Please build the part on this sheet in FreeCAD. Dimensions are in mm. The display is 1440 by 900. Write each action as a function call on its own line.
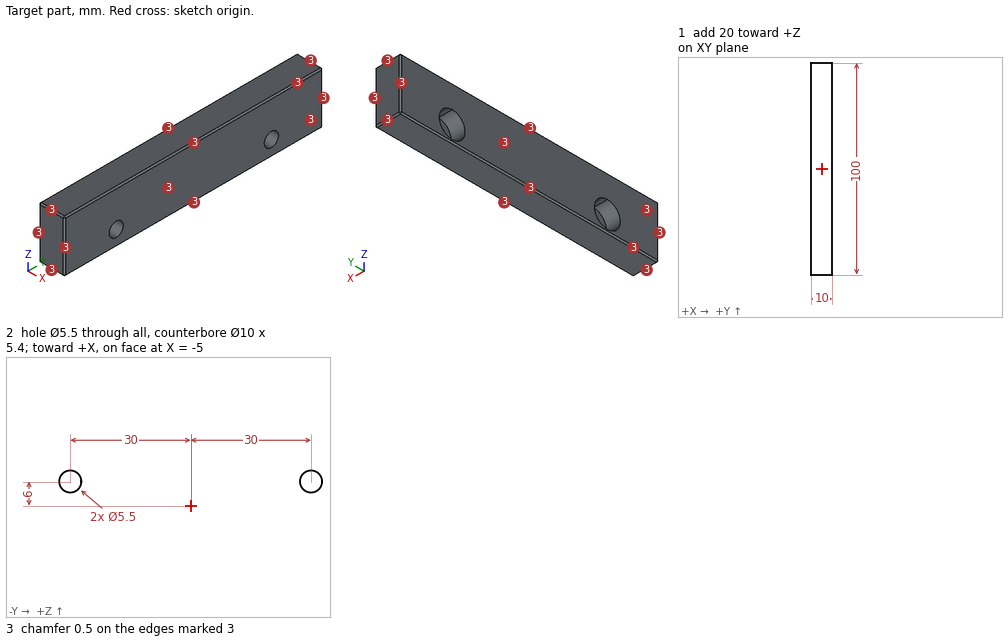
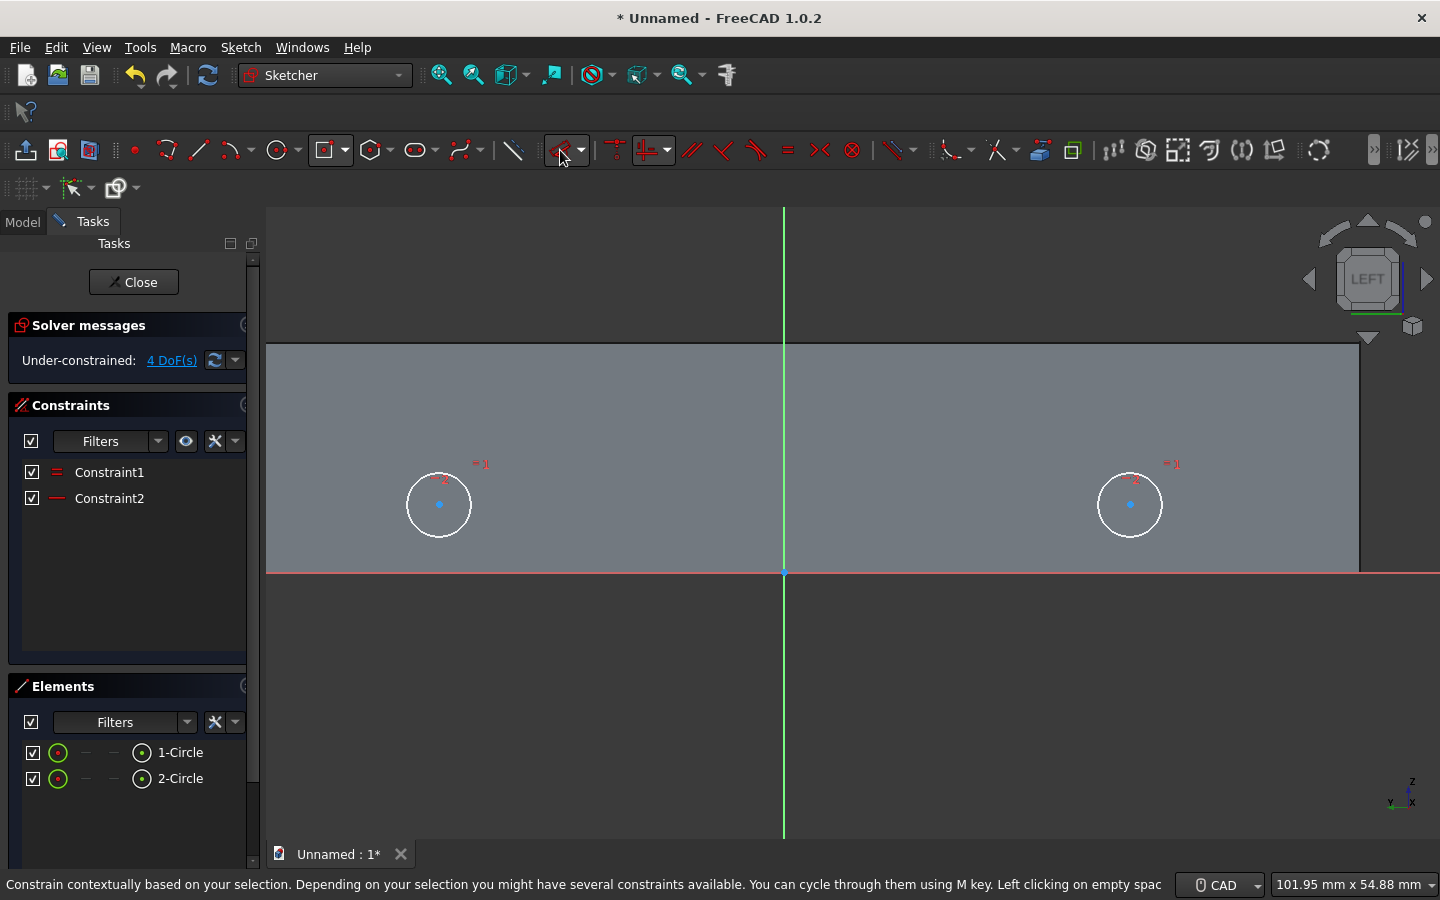
click(461, 482)
click(483, 459)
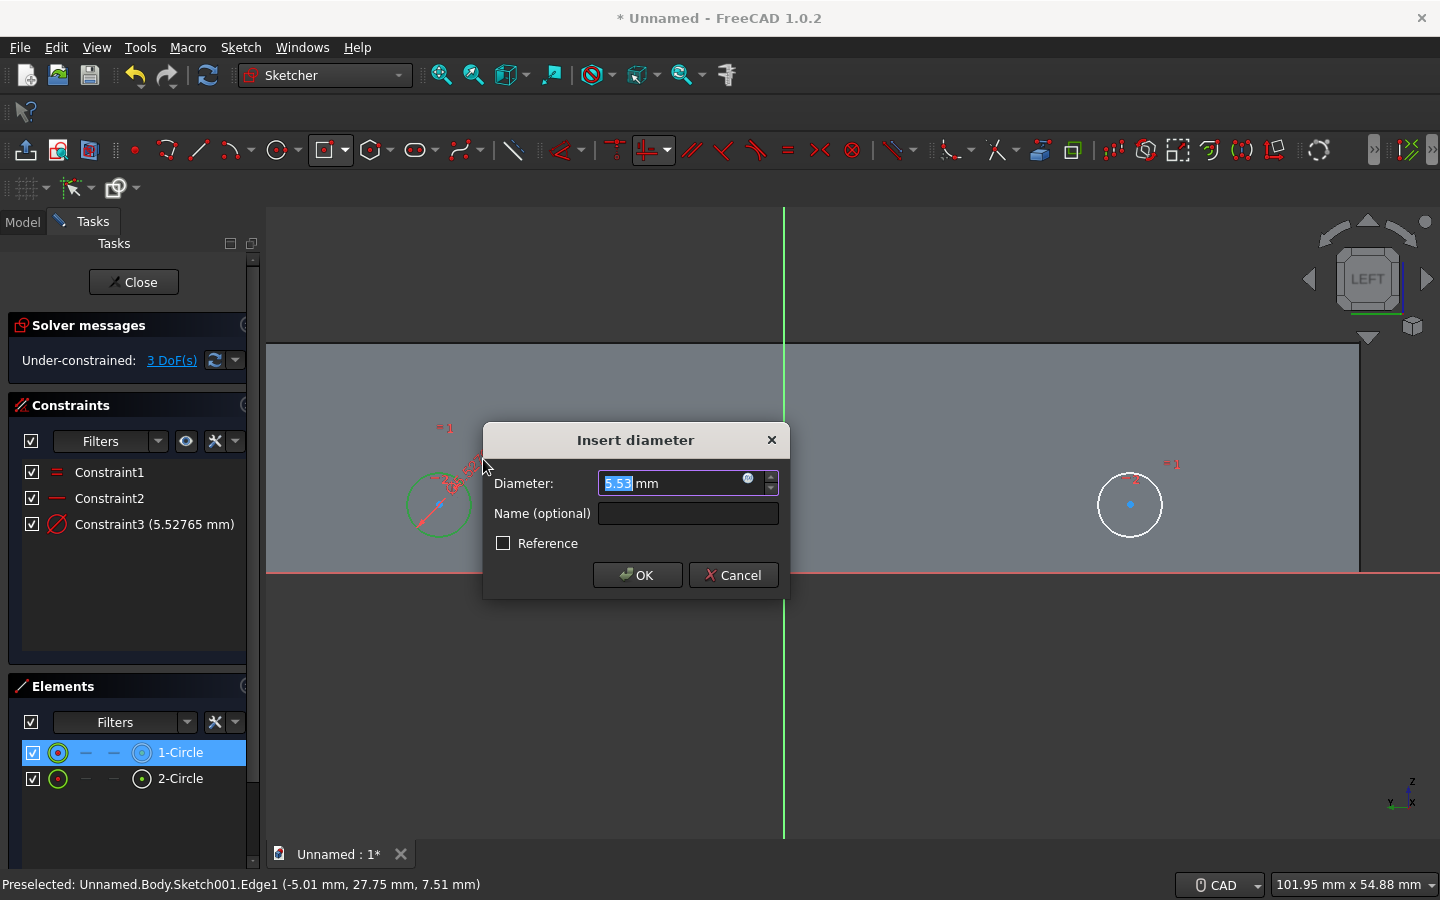
text(5.5)
key(Return)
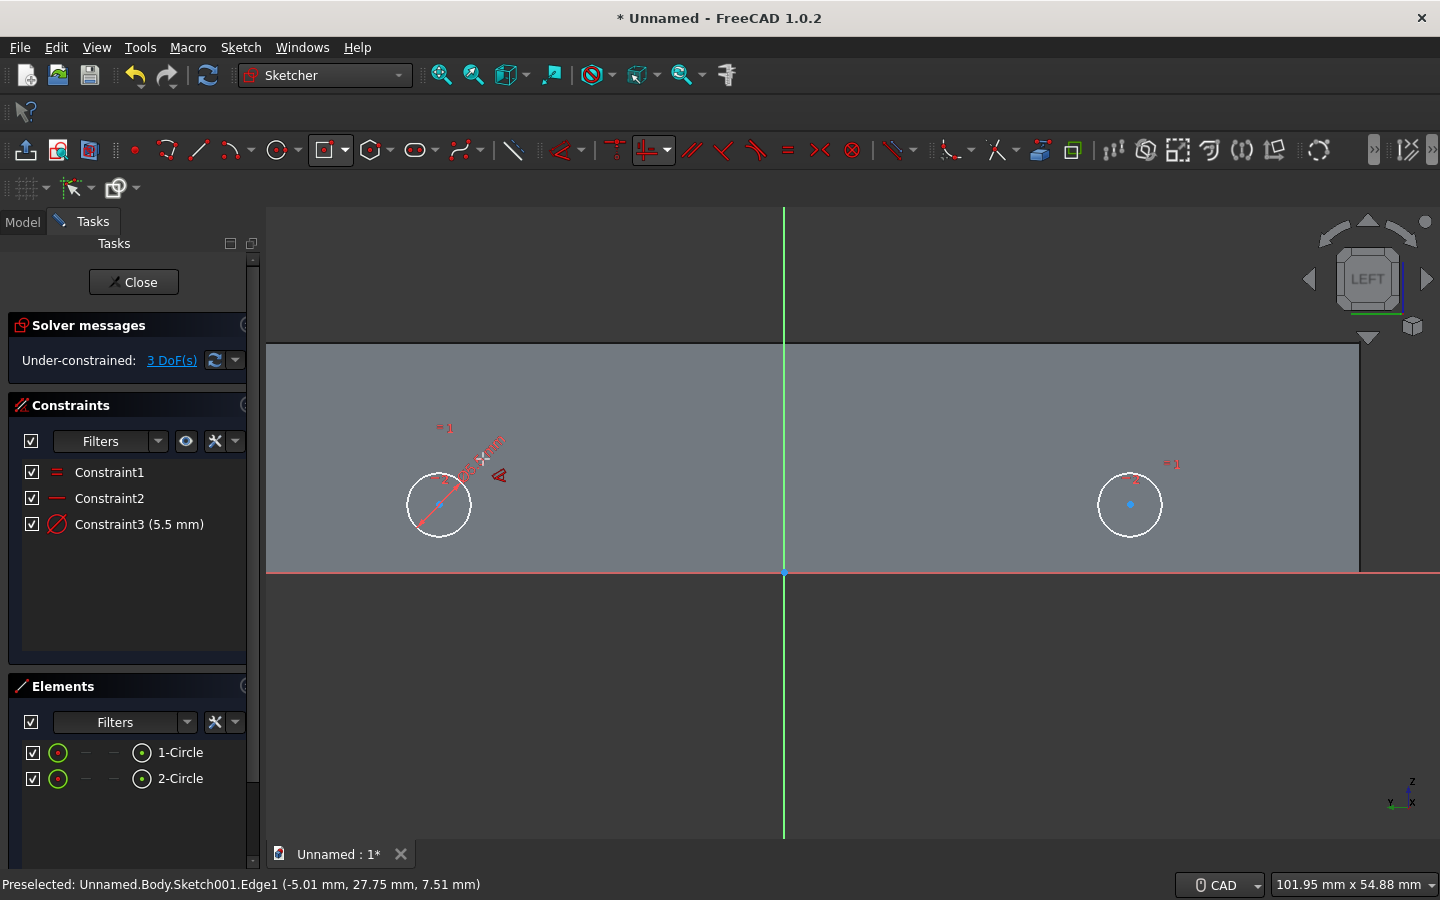
click(439, 505)
click(405, 539)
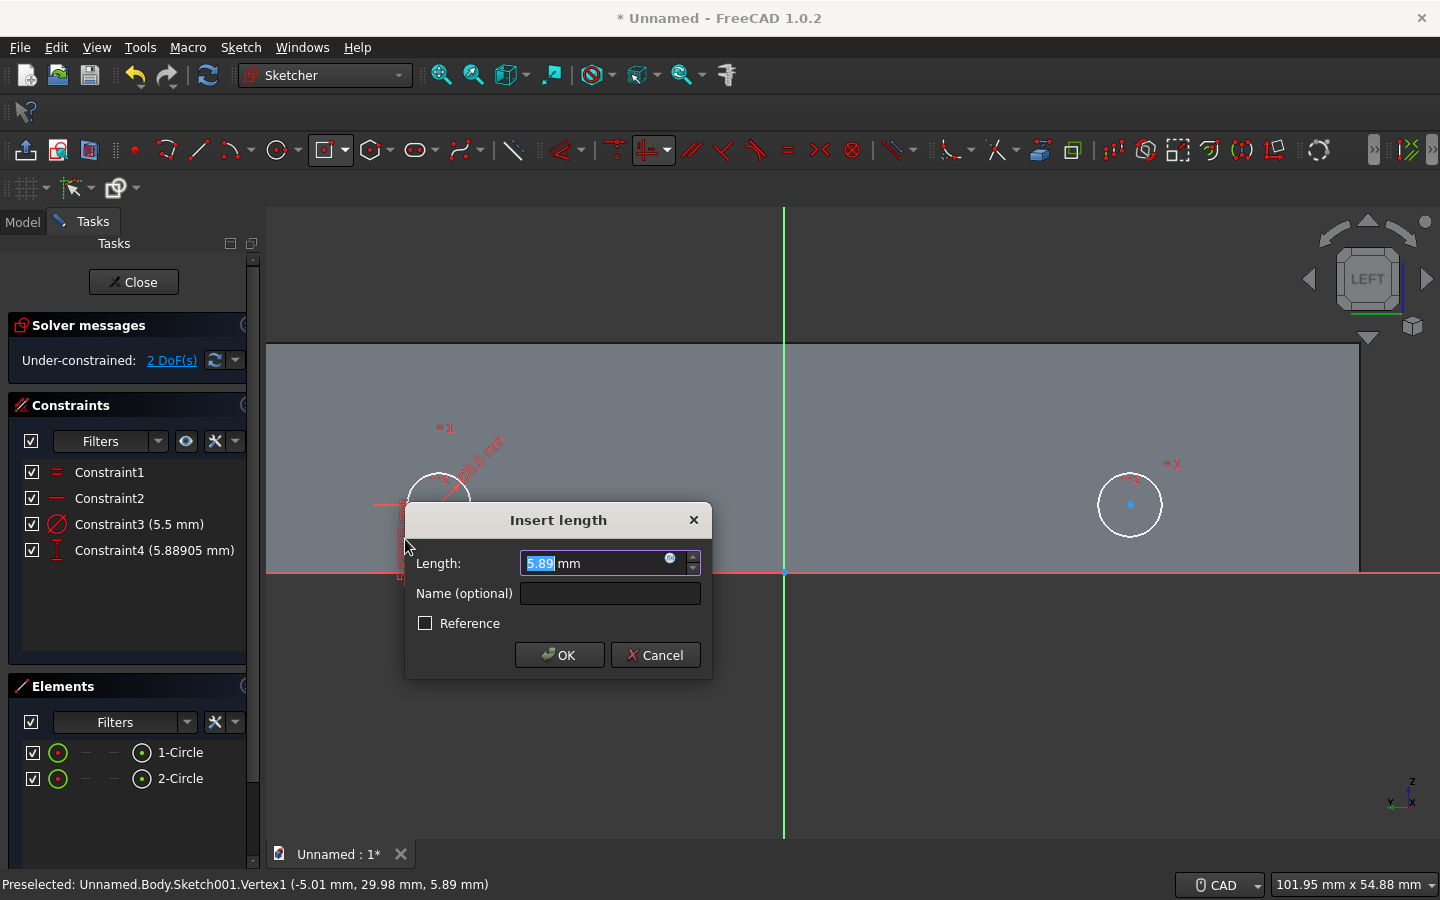
text(6)
key(Return)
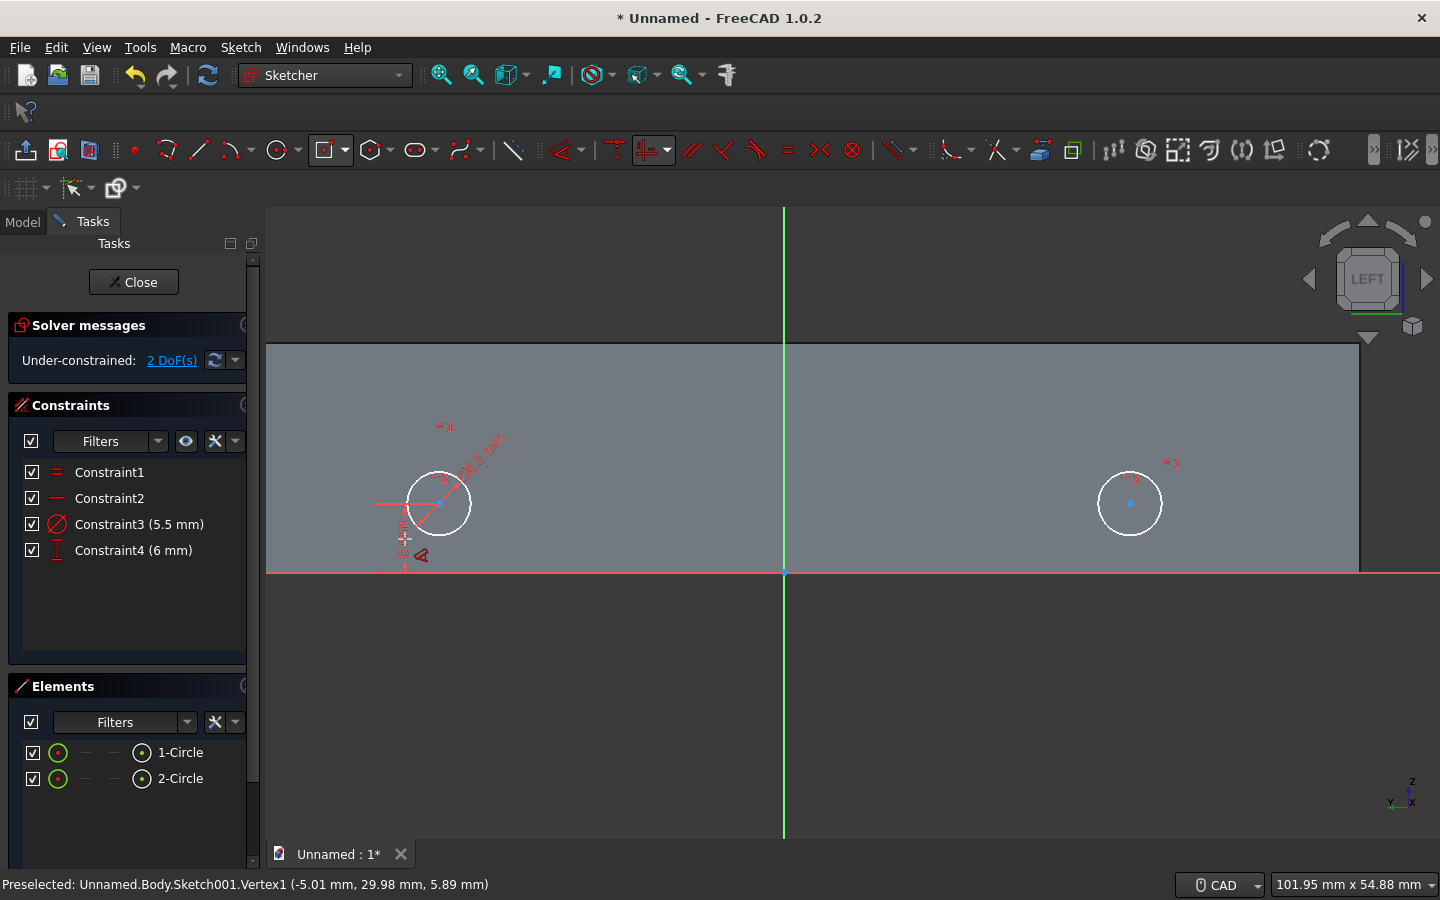
click(439, 504)
click(612, 607)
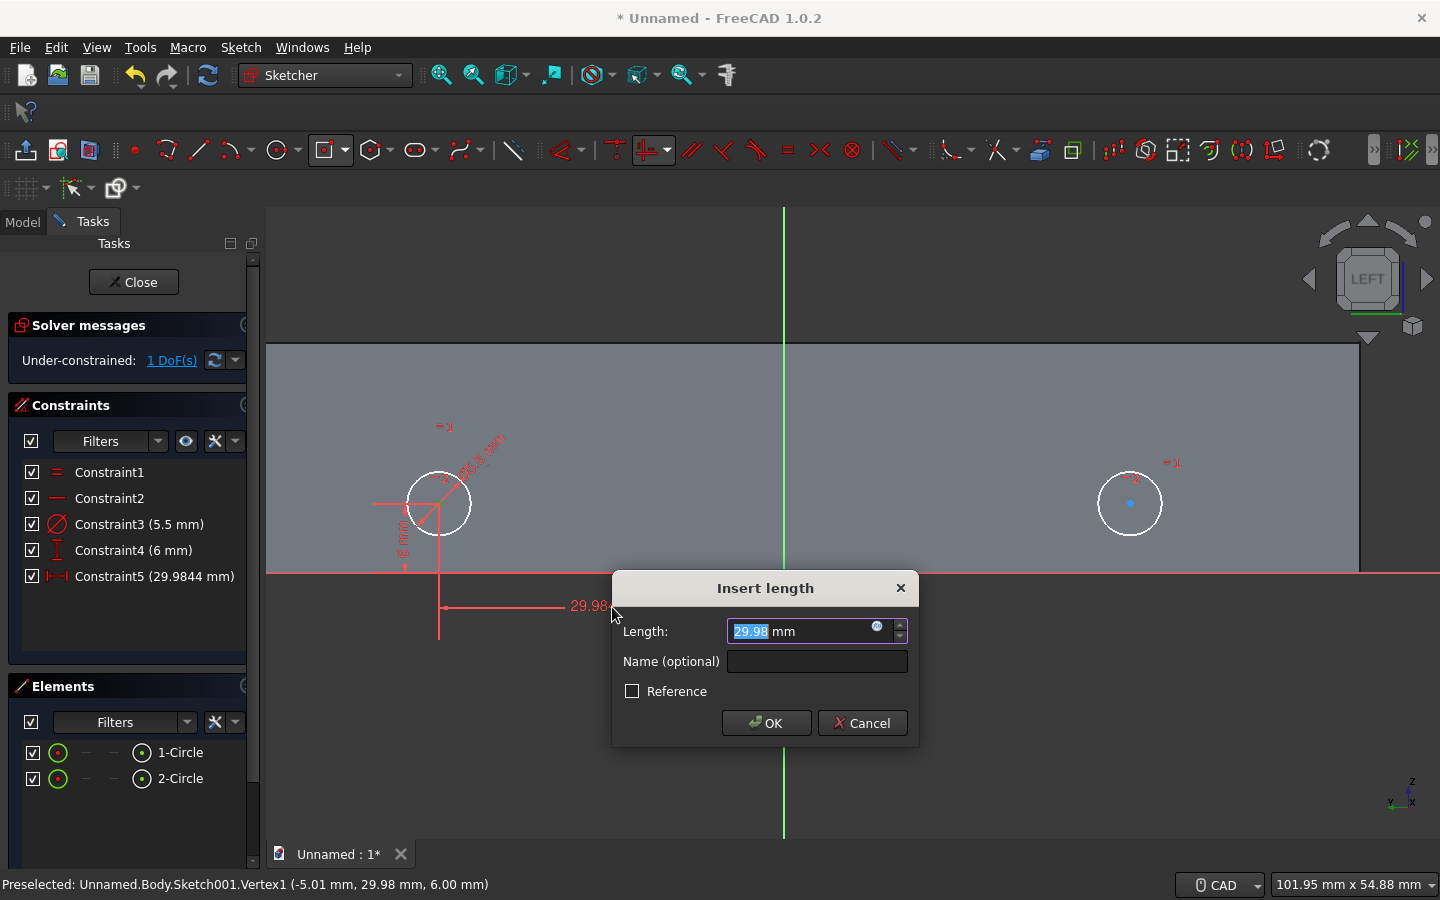
text(30)
key(Return)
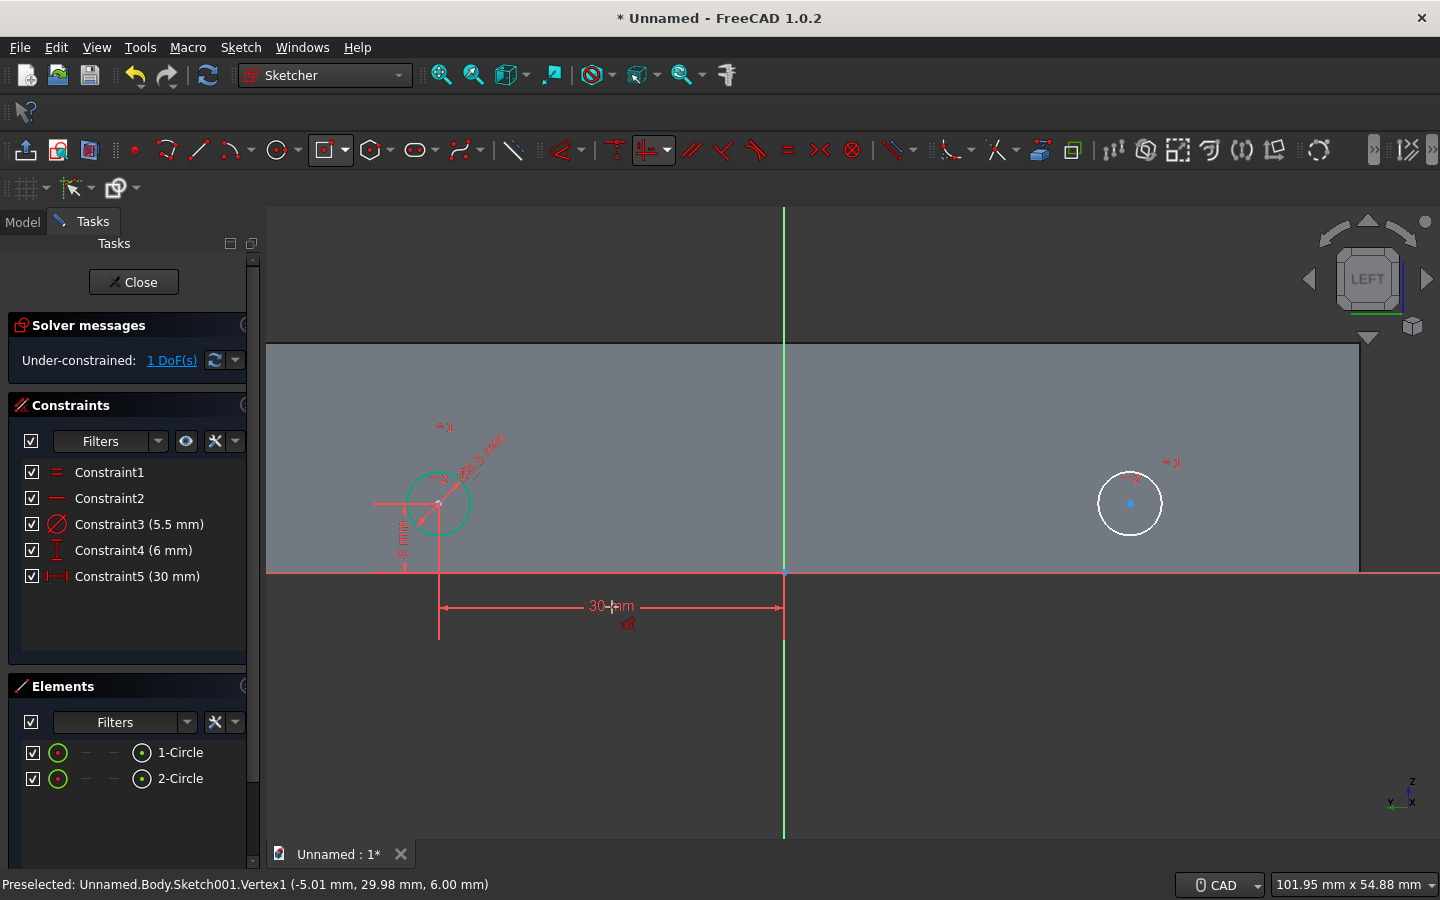
click(1130, 504)
click(957, 607)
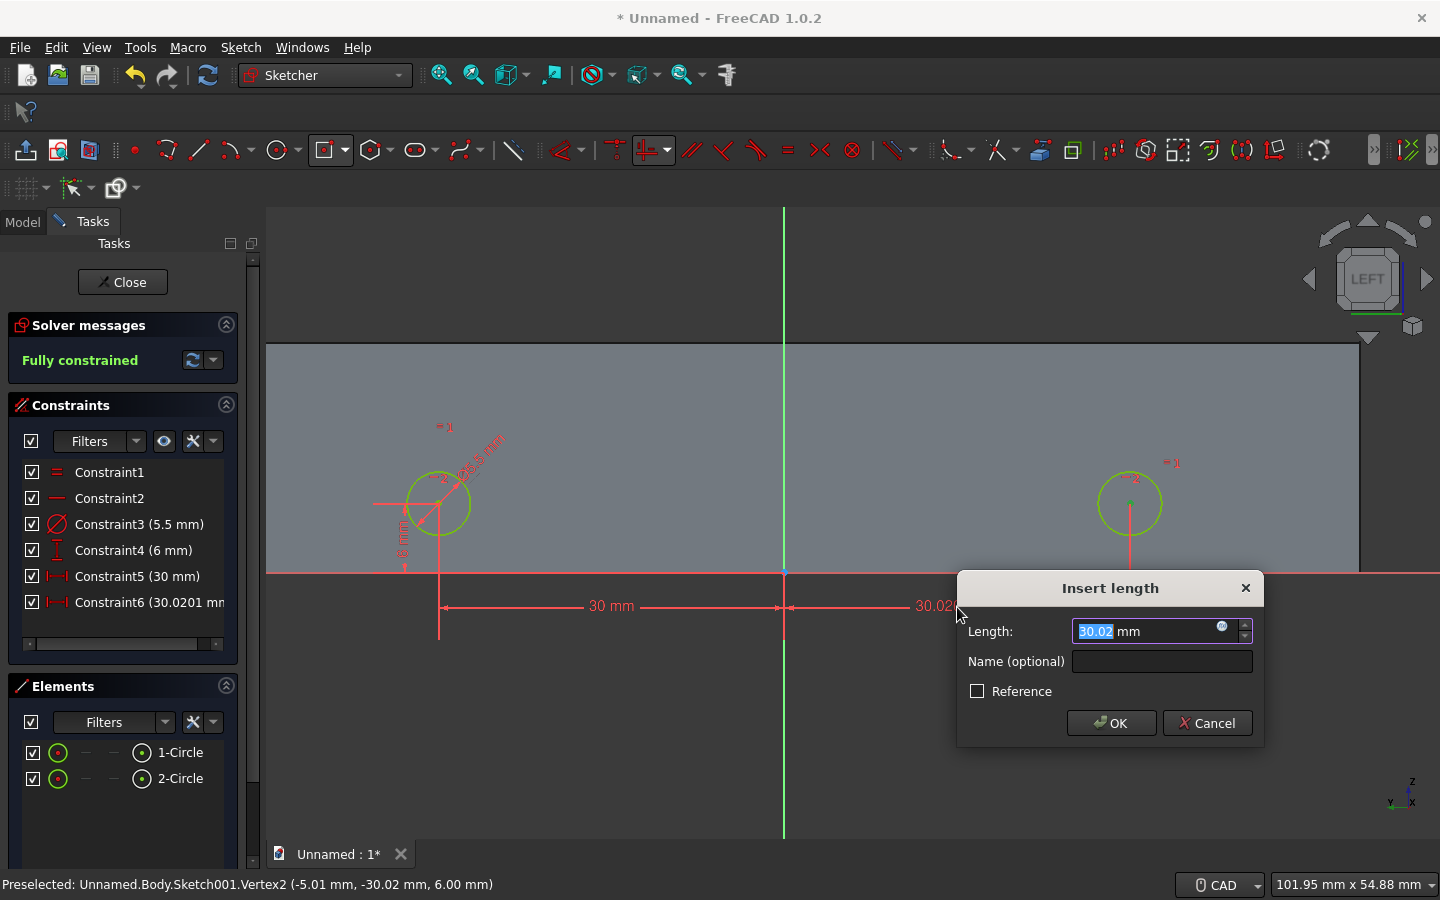
text(30)
key(Return)
key(Escape)